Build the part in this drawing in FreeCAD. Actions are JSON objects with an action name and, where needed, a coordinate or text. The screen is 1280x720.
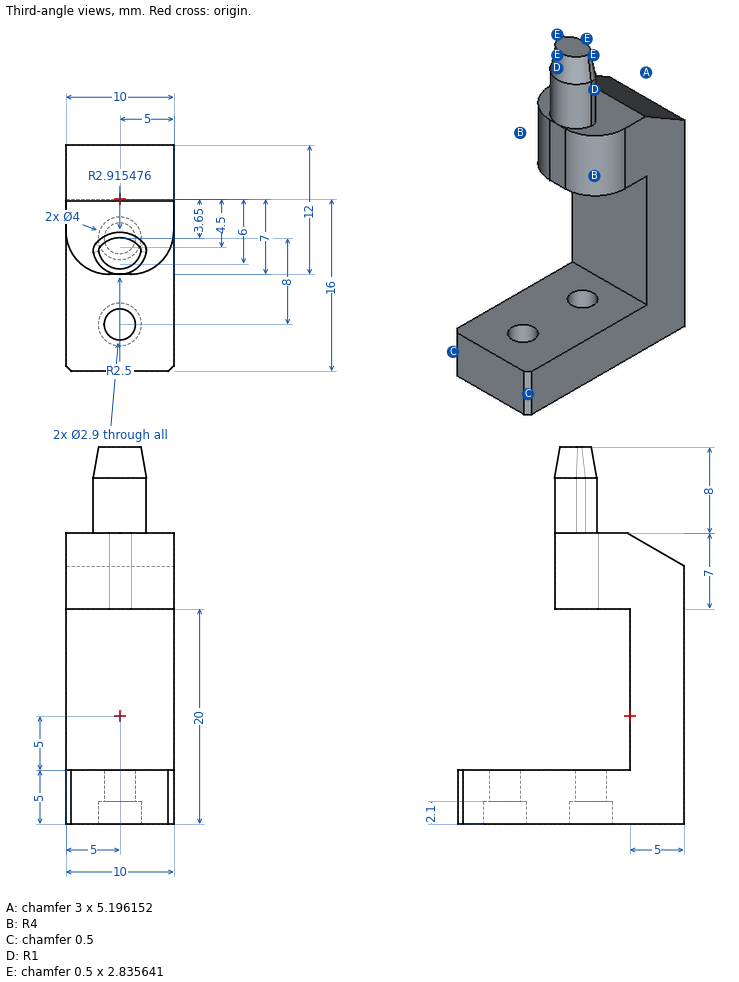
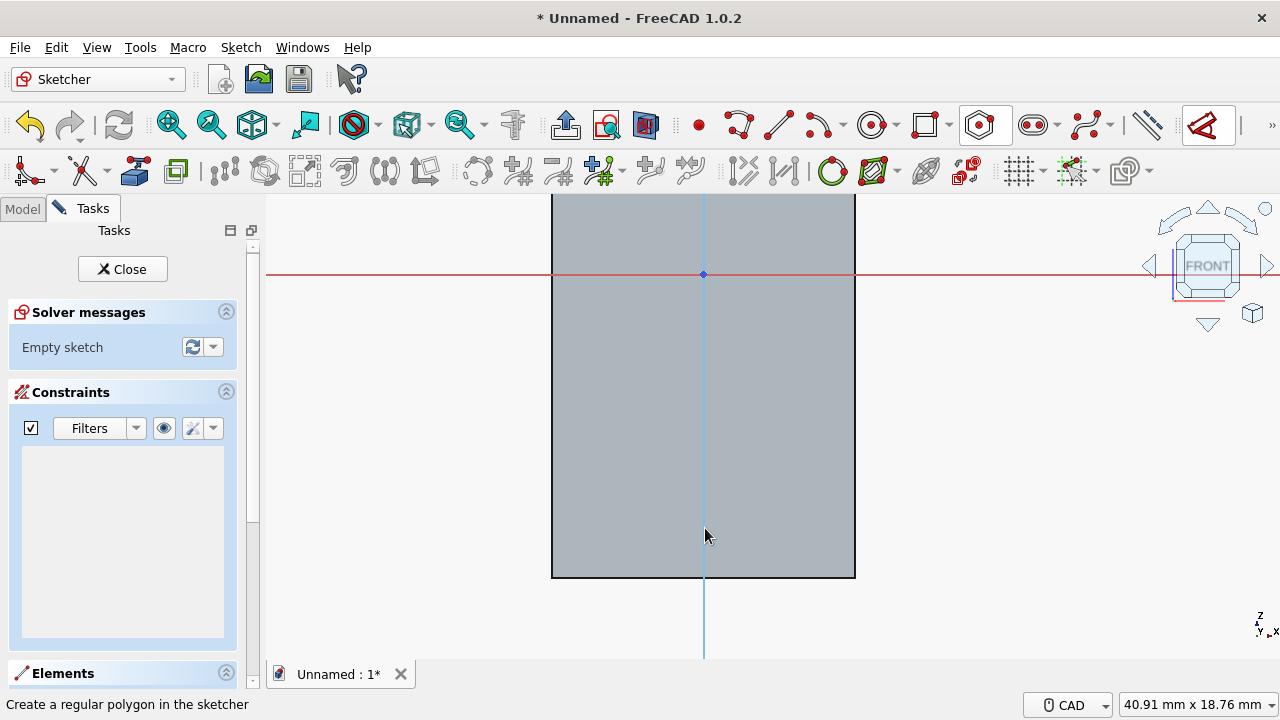
{"action": "key", "text": "g r"}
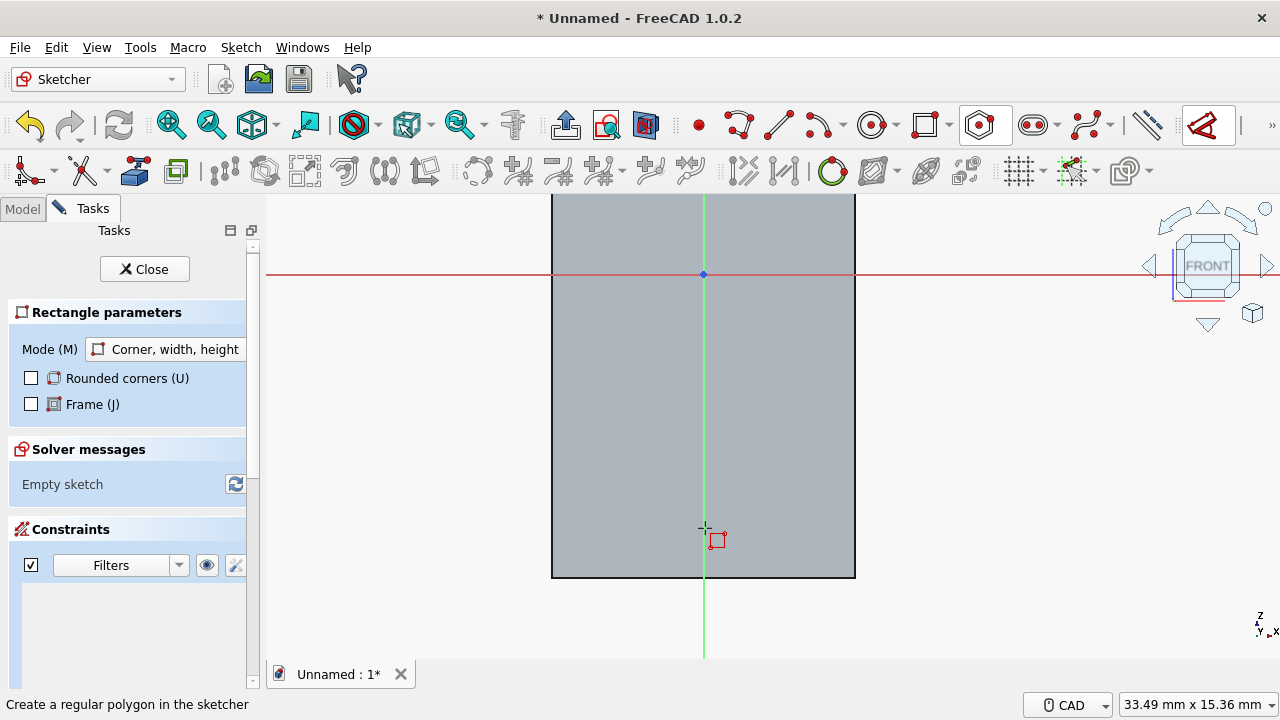
{"action": "left_click", "coordinate": [552, 426]}
{"action": "left_click", "coordinate": [855, 578]}
{"action": "key", "text": "Escape"}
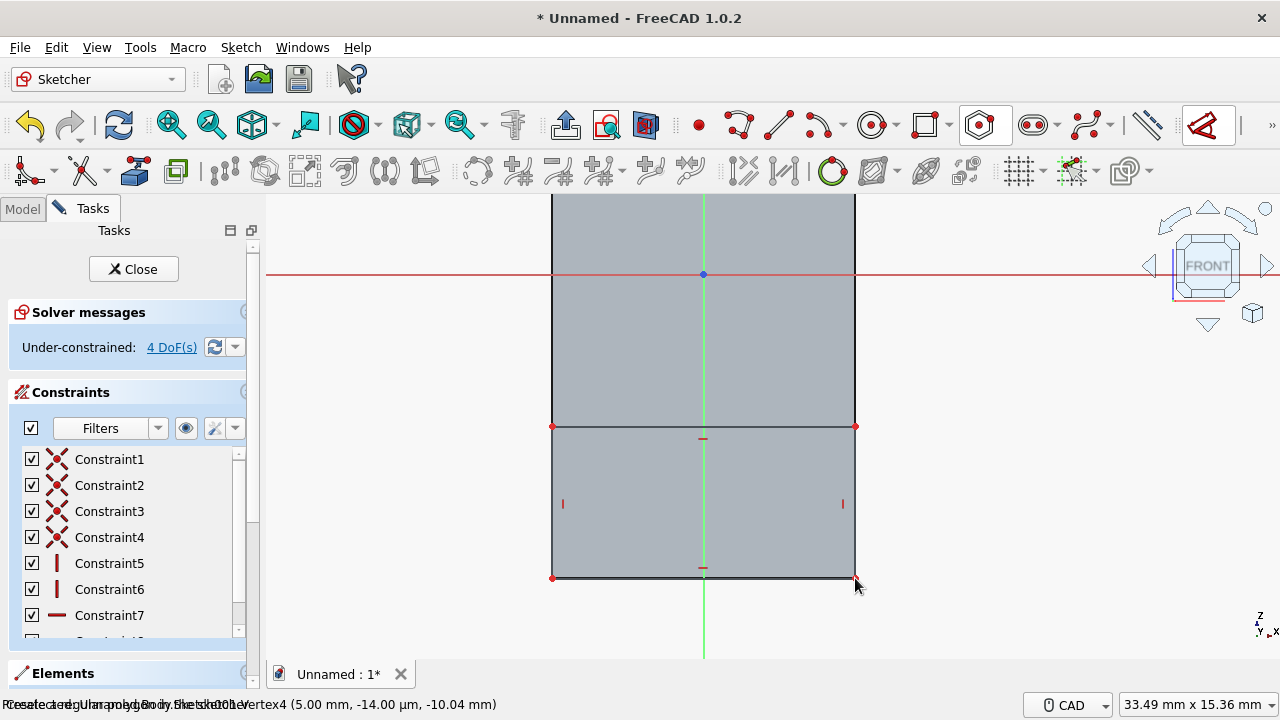
{"action": "key", "text": "d"}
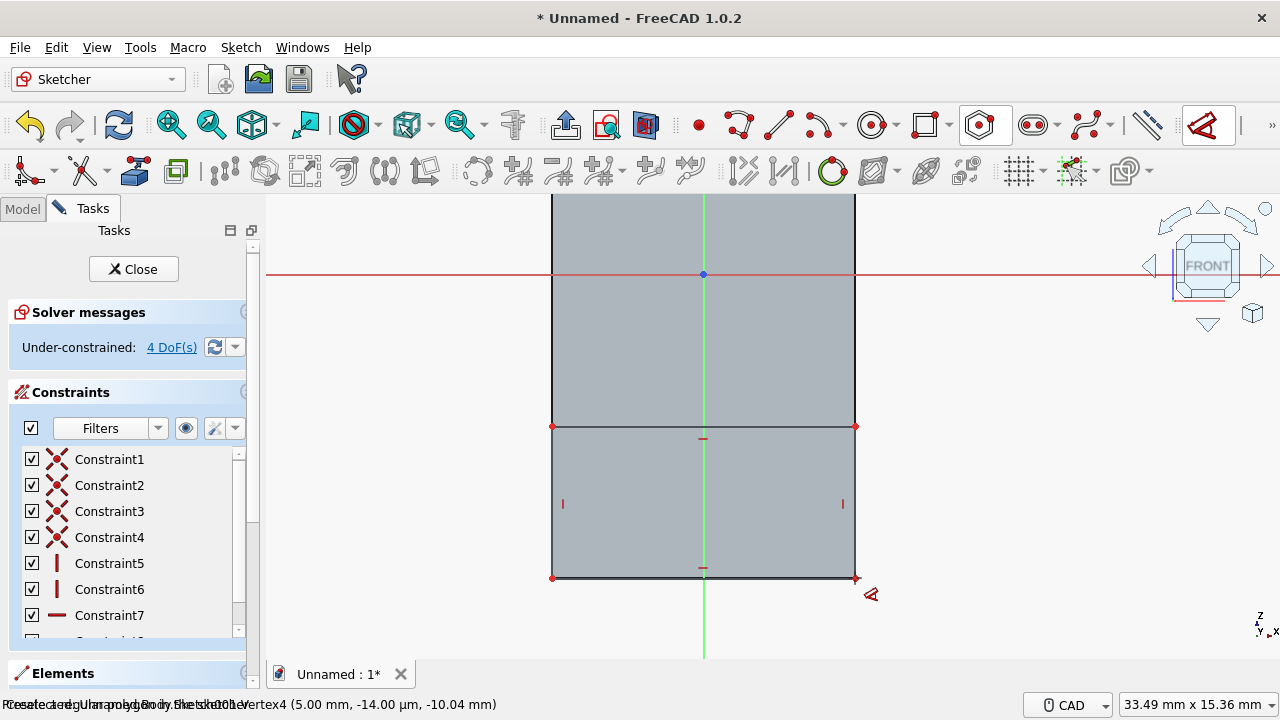
{"action": "left_click", "coordinate": [552, 473]}
{"action": "left_click", "coordinate": [518, 503]}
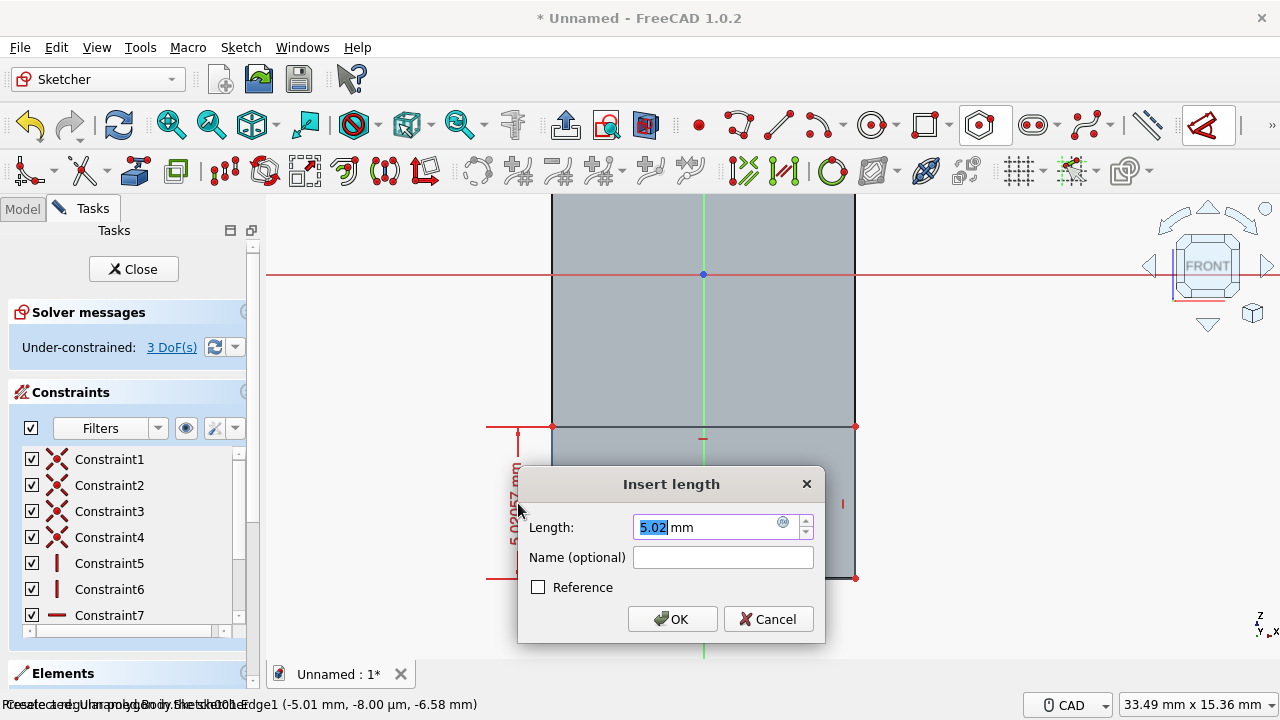
{"action": "type", "text": "5"}
{"action": "key", "text": "Return"}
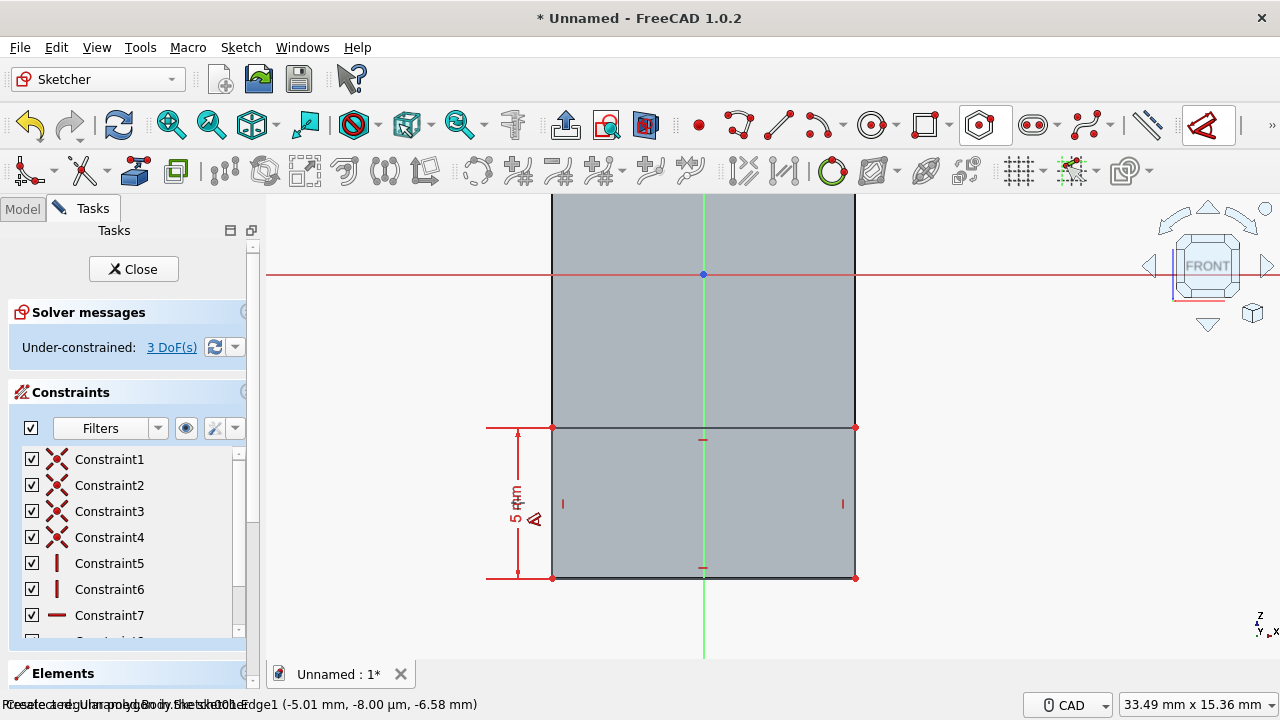
{"action": "left_click", "coordinate": [643, 579]}
{"action": "left_click", "coordinate": [634, 613]}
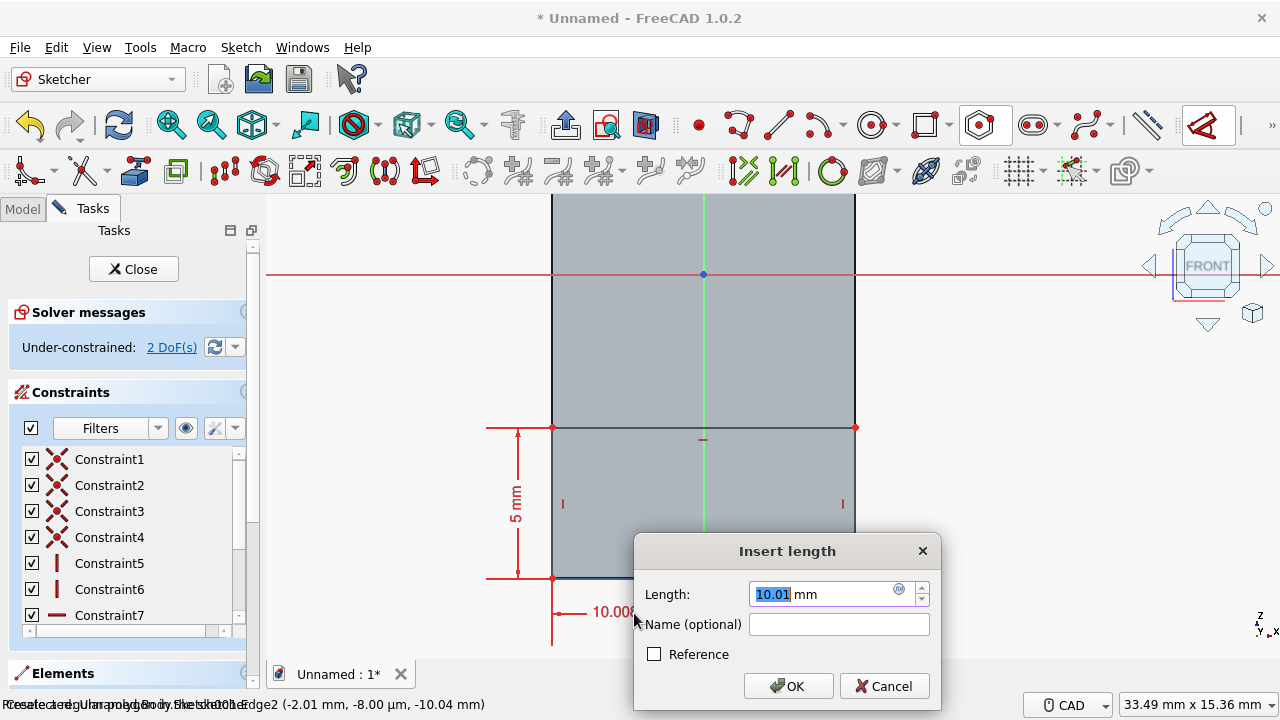
{"action": "type", "text": "10"}
{"action": "key", "text": "Return"}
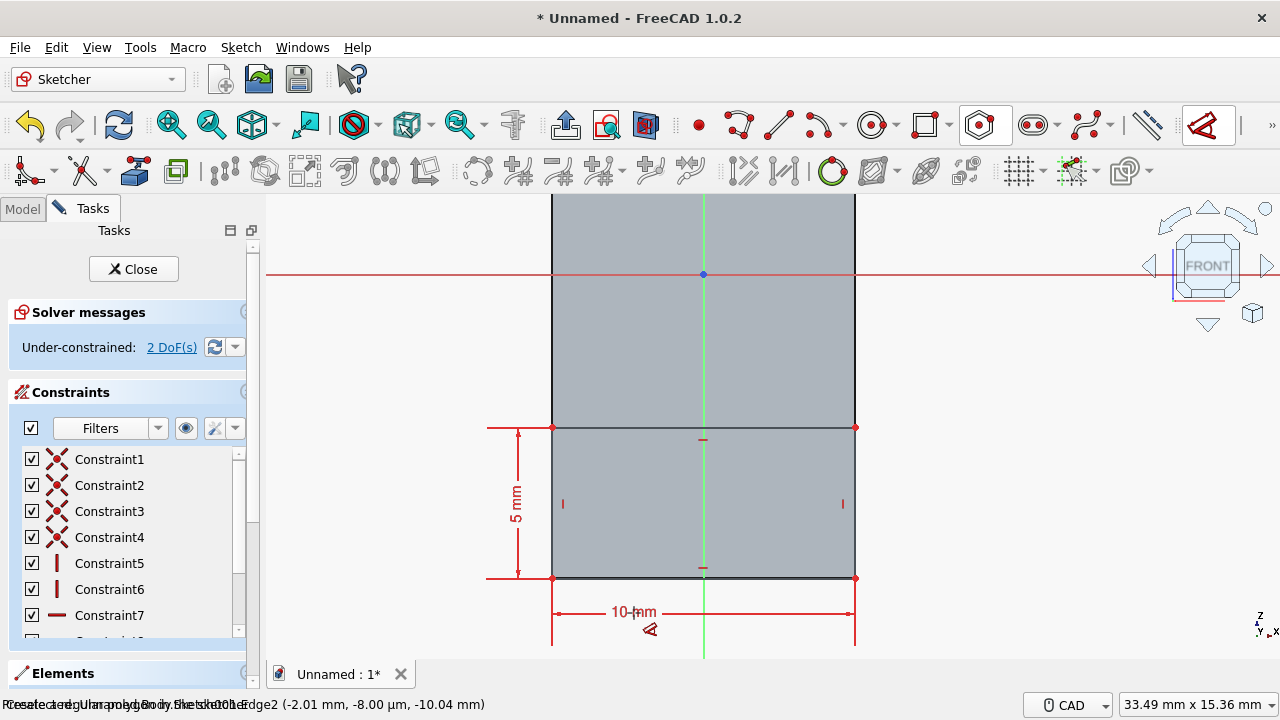
{"action": "left_click", "coordinate": [552, 428]}
{"action": "left_click", "coordinate": [628, 241]}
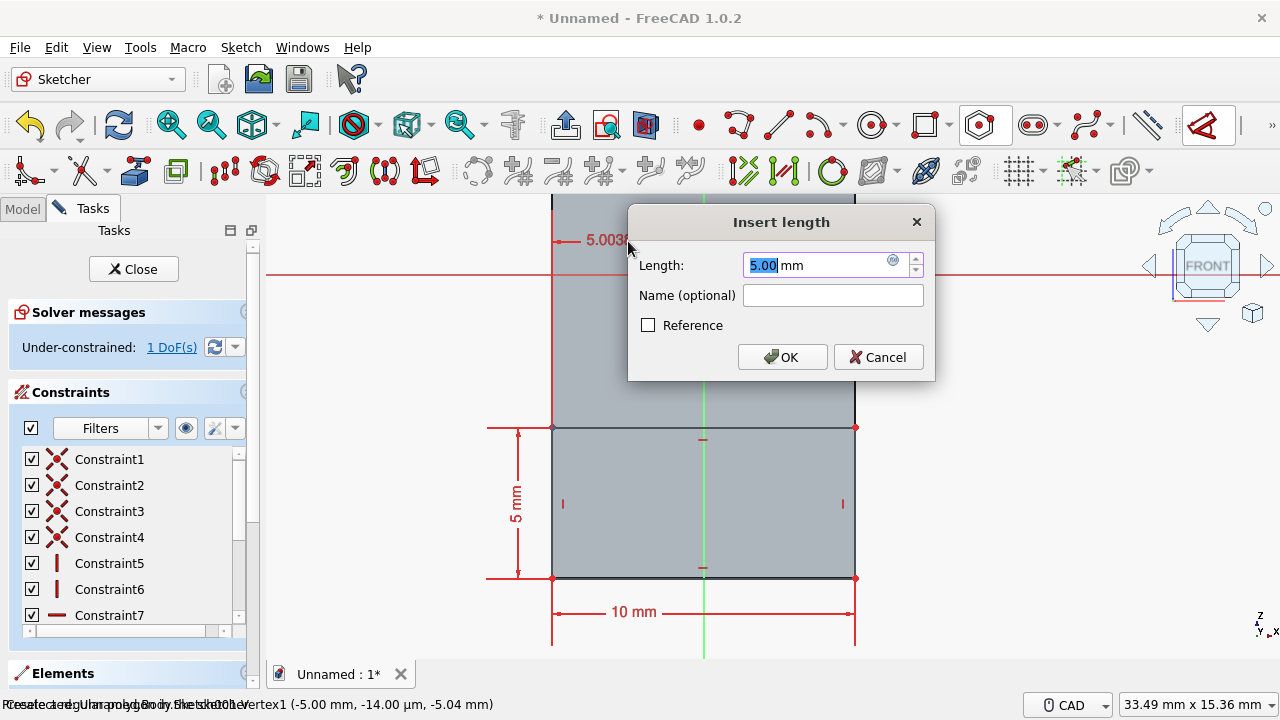
{"action": "type", "text": "5"}
{"action": "key", "text": "Return"}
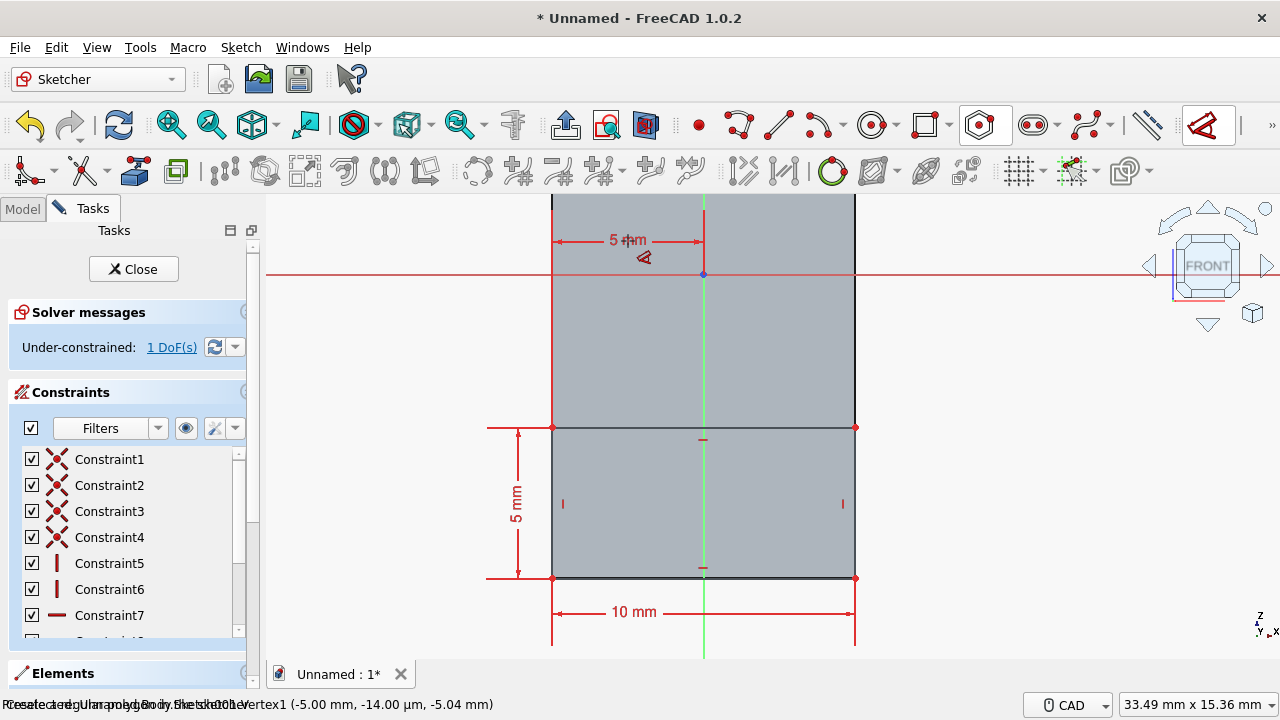
{"action": "left_click", "coordinate": [552, 428]}
{"action": "left_click", "coordinate": [518, 351]}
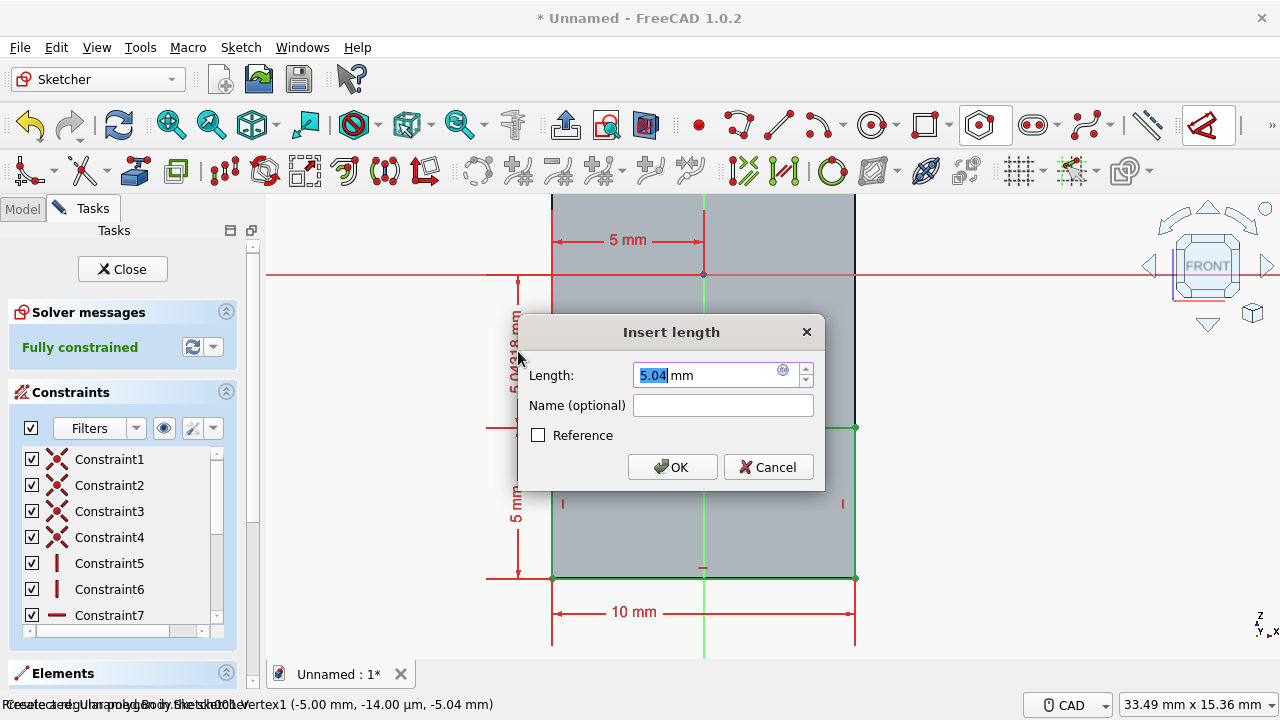
{"action": "type", "text": "5"}
{"action": "key", "text": "Return"}
{"action": "key", "text": "Escape"}